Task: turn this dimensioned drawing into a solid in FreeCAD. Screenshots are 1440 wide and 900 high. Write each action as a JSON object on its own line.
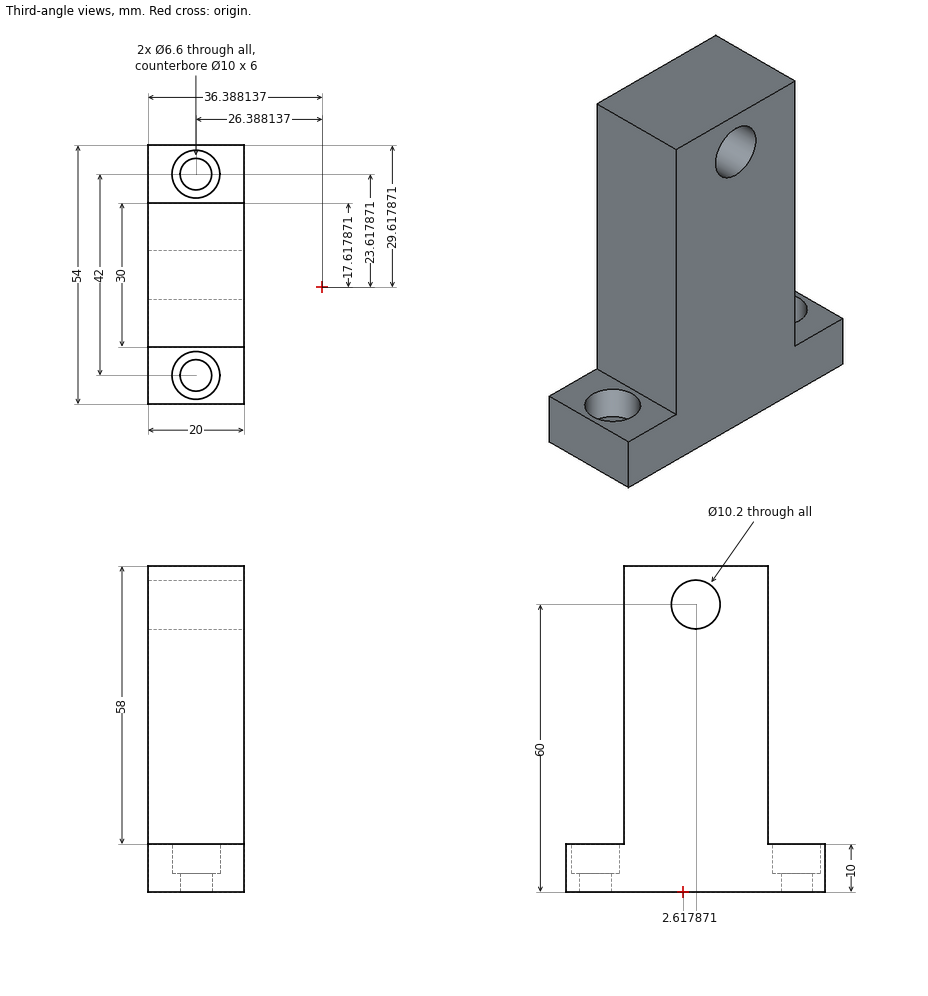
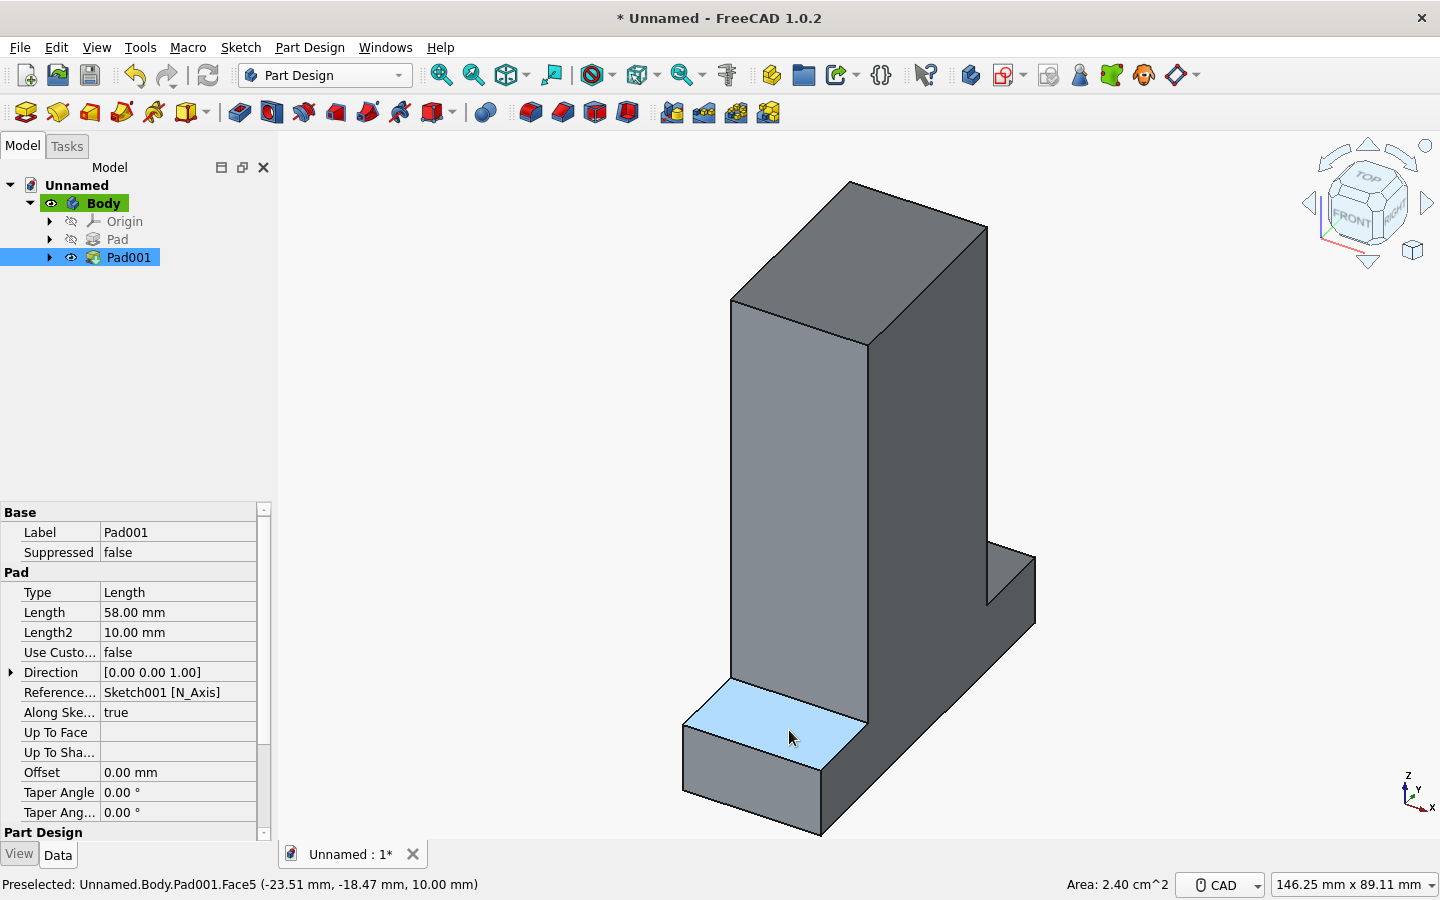
{"action": "left_click", "coordinate": [1004, 76]}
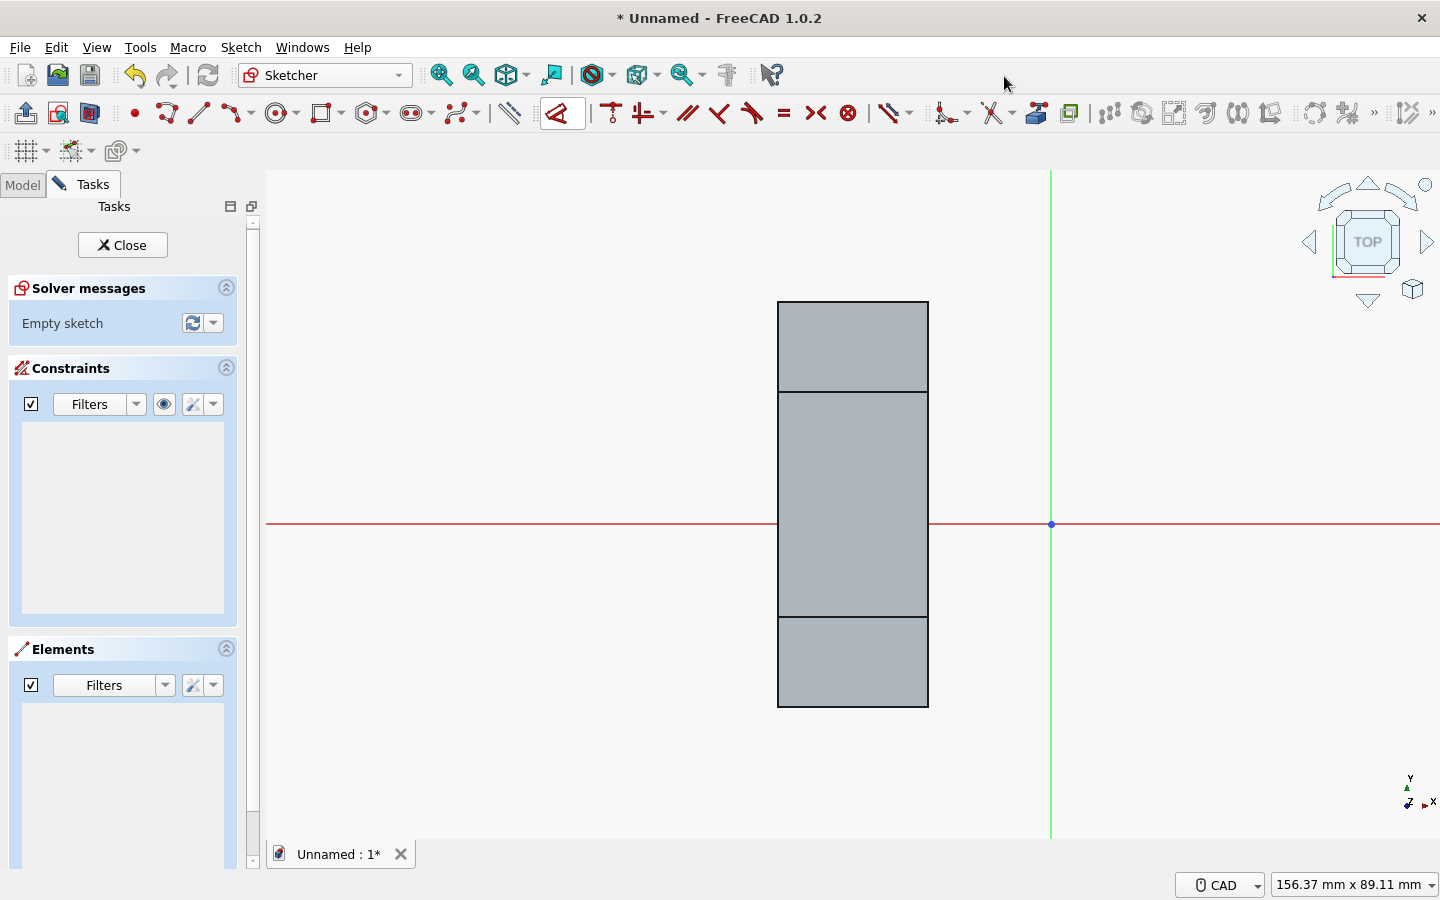
{"action": "left_click", "coordinate": [276, 114]}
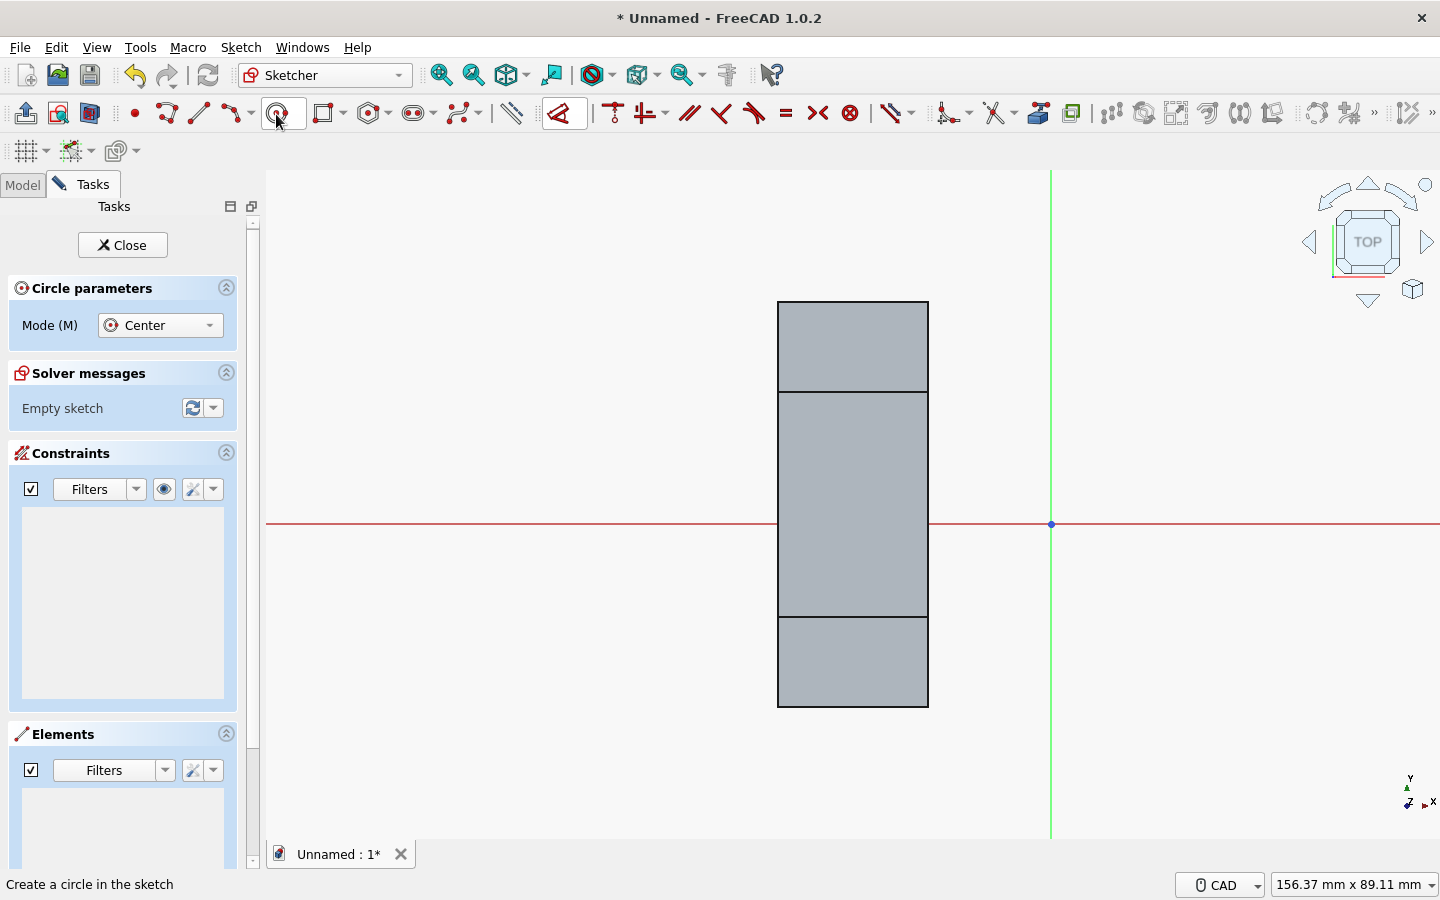
{"action": "left_click", "coordinate": [853, 347]}
{"action": "left_click", "coordinate": [871, 329]}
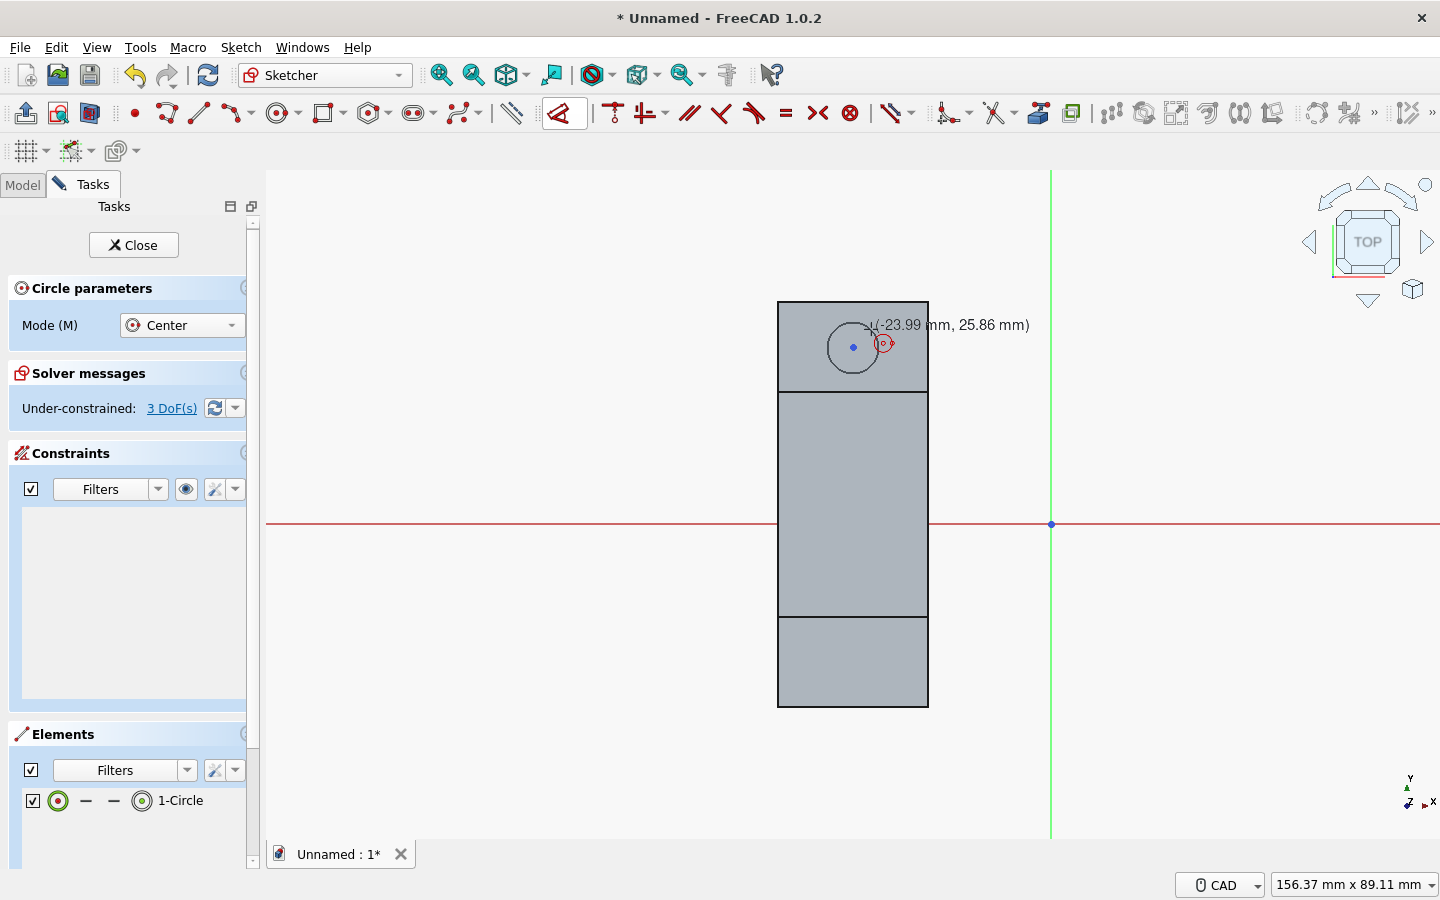
{"action": "left_click", "coordinate": [853, 662]}
{"action": "left_click", "coordinate": [871, 645]}
{"action": "key", "text": "Escape"}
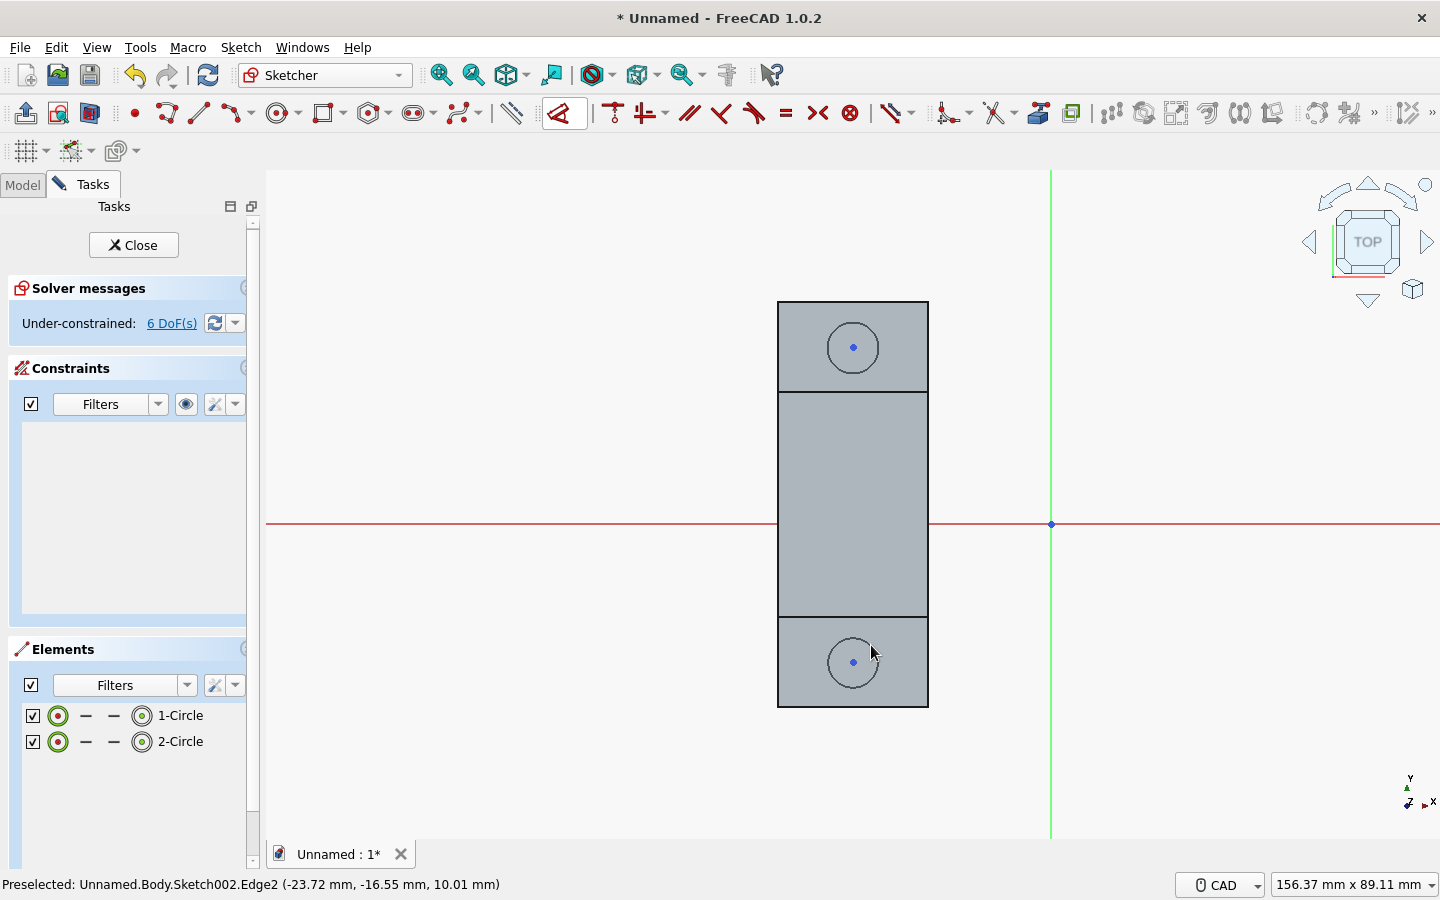
{"action": "left_click", "coordinate": [871, 330]}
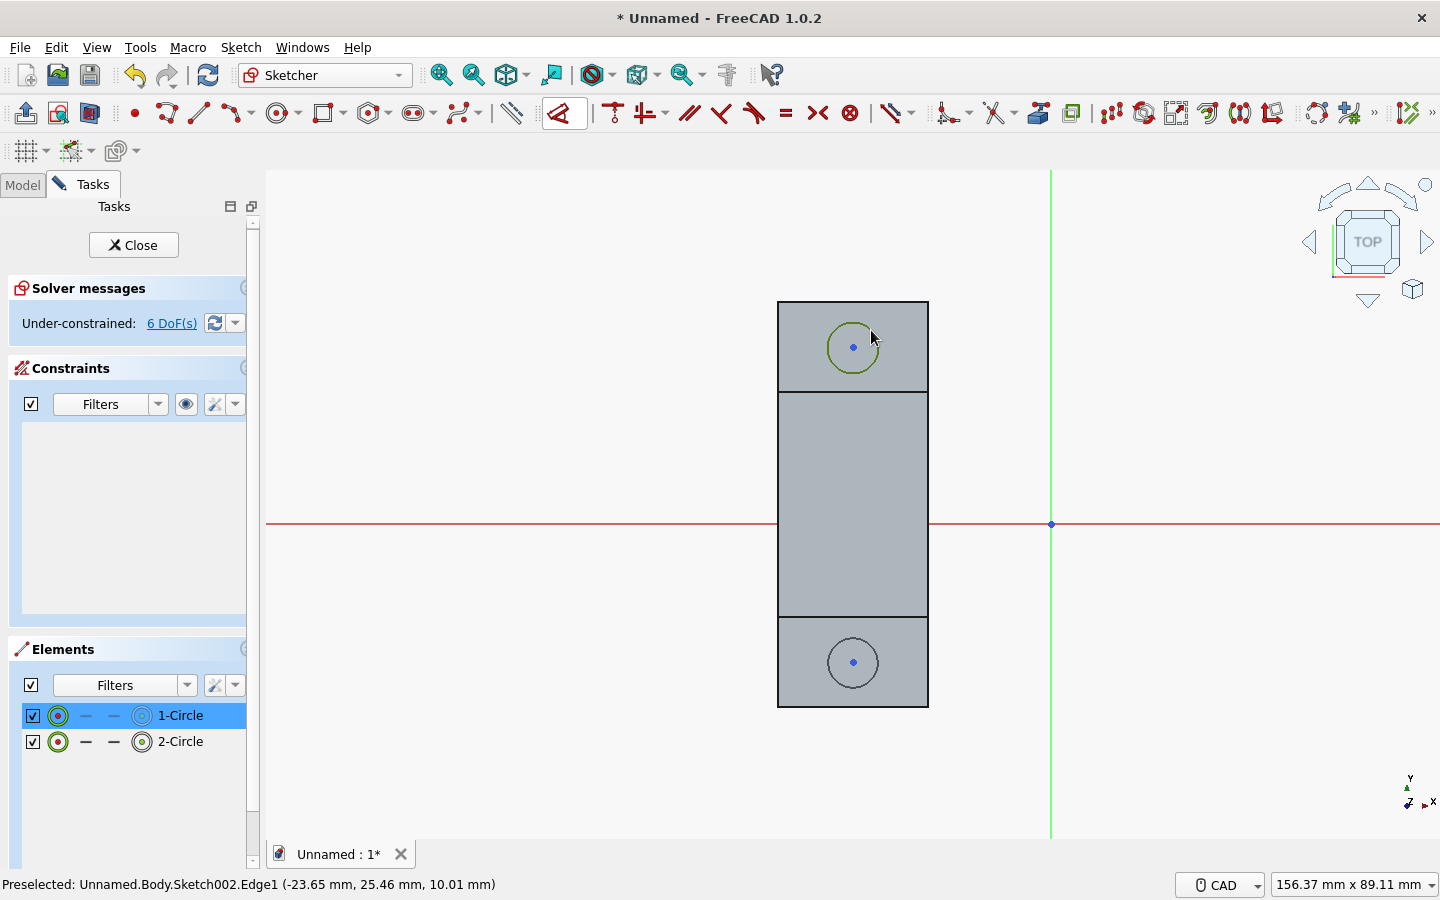
{"action": "left_click", "coordinate": [870, 645]}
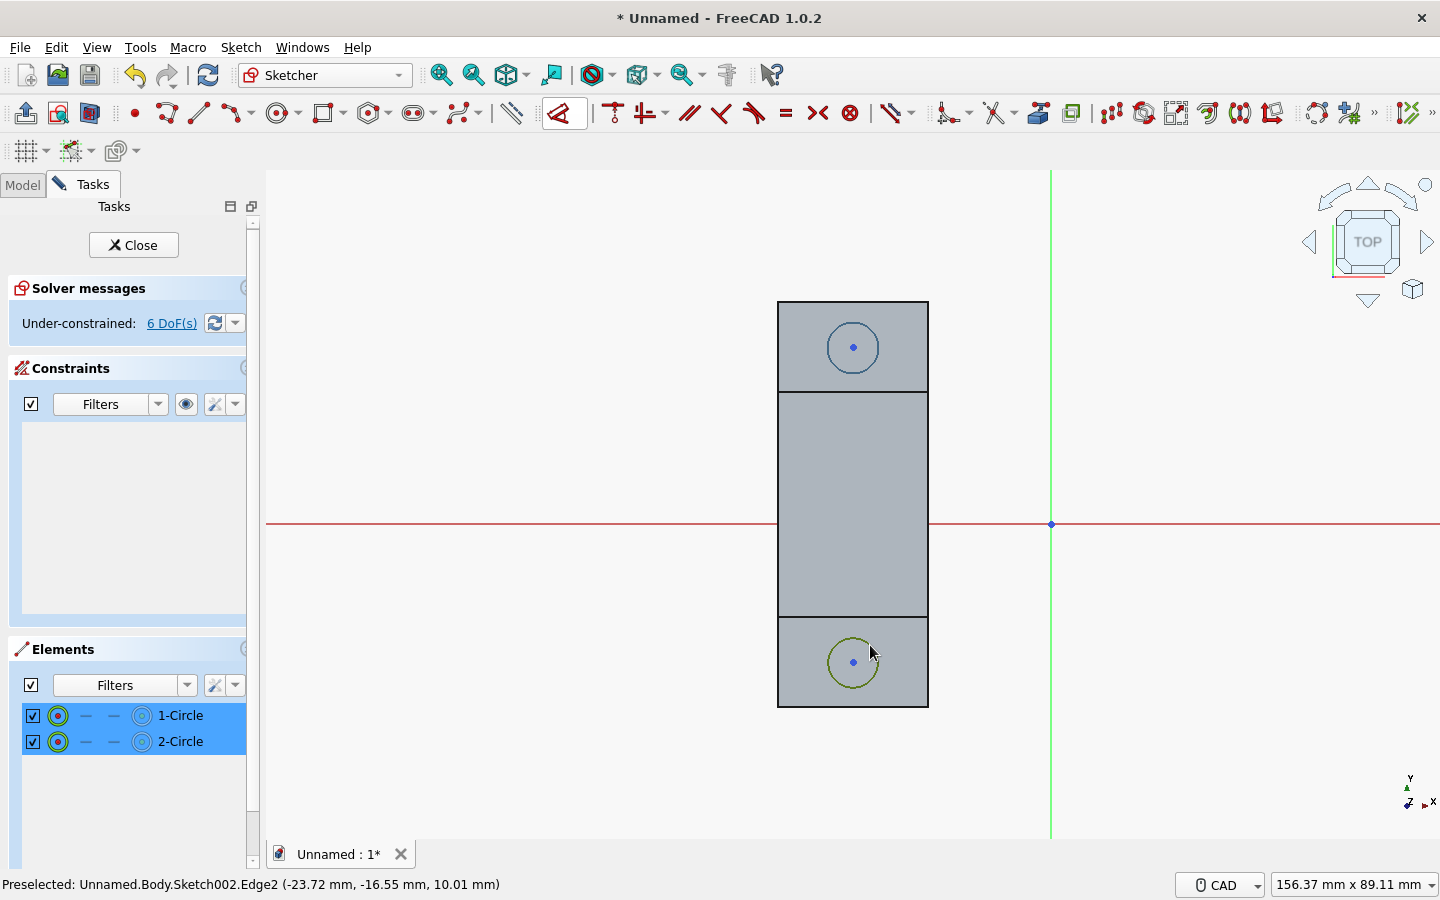
{"action": "left_click", "coordinate": [786, 114]}